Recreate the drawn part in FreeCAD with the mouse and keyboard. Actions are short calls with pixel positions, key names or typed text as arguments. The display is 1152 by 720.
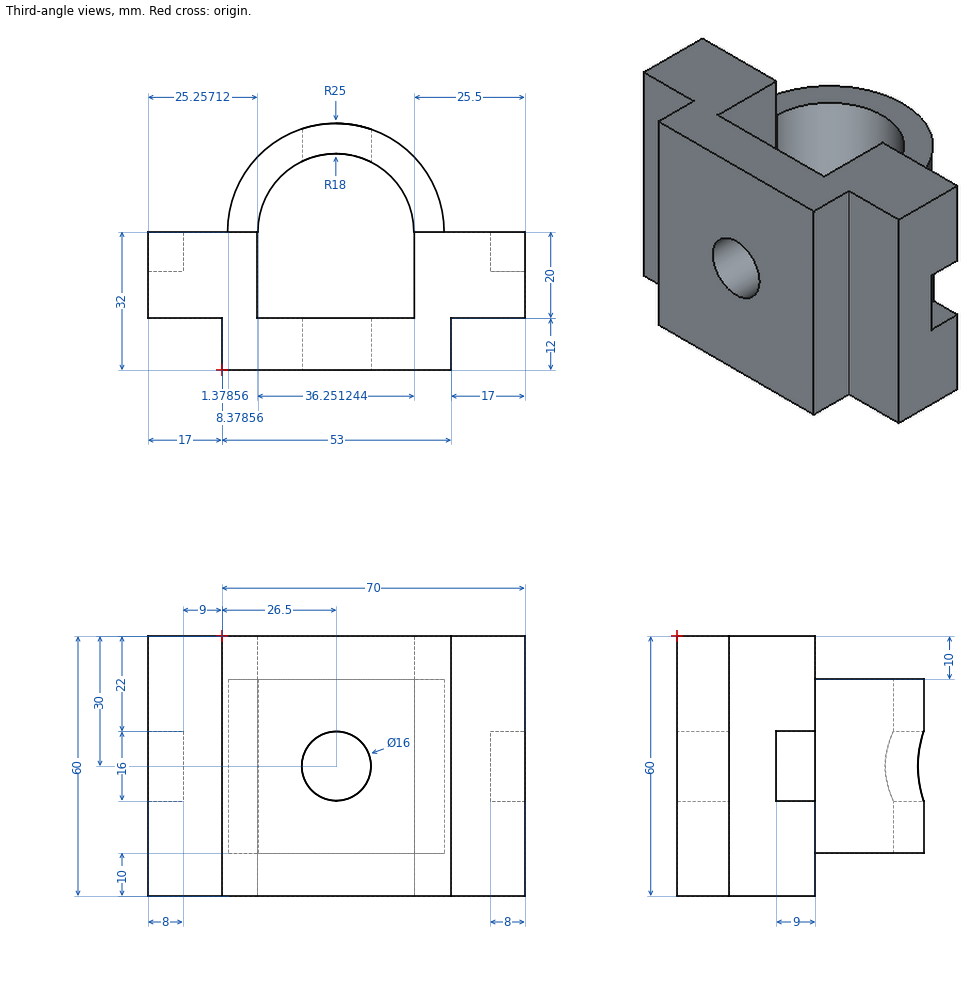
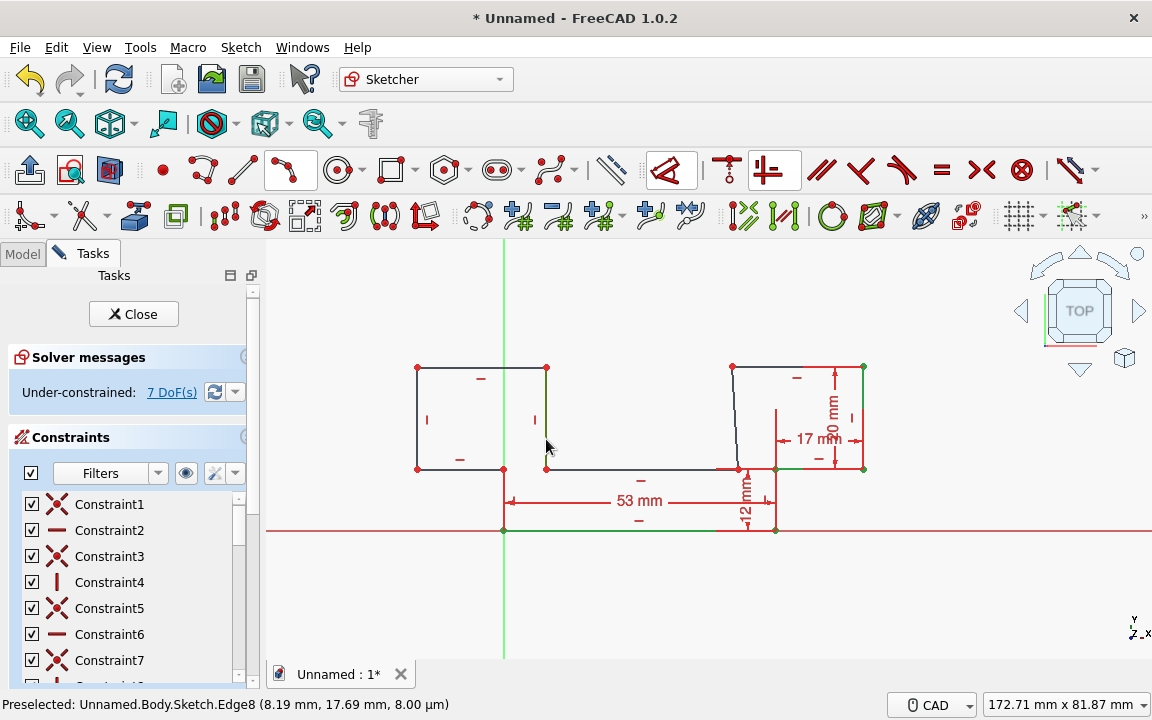
click(692, 170)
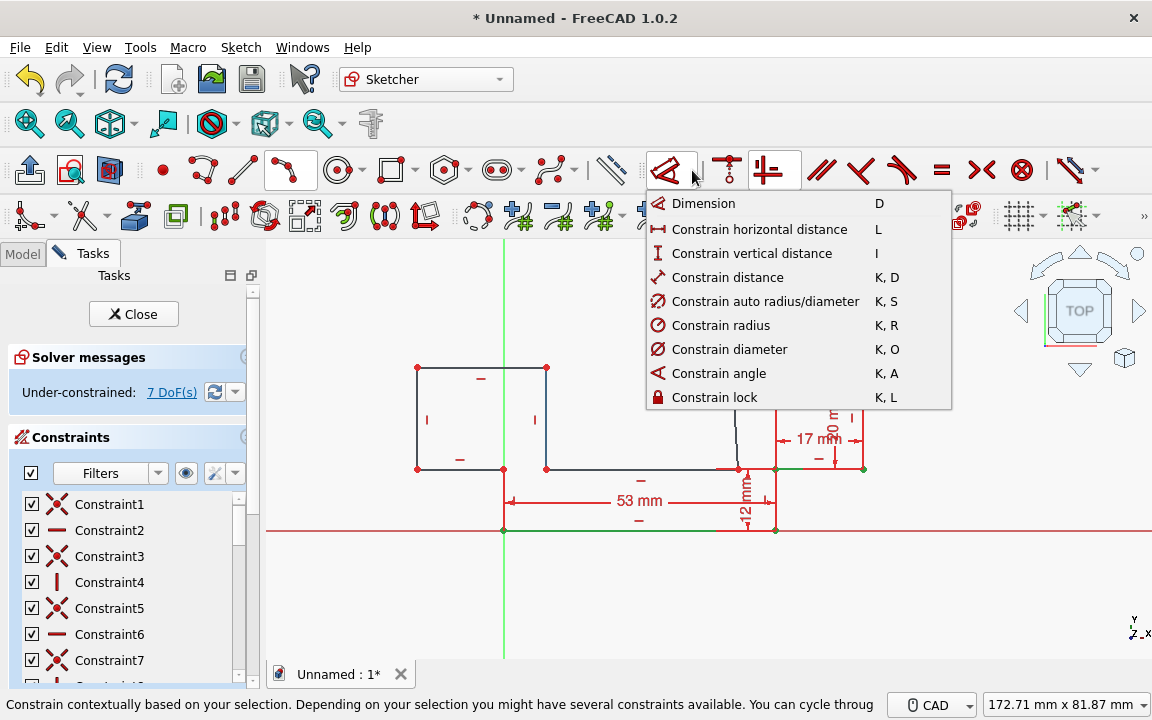
click(799, 253)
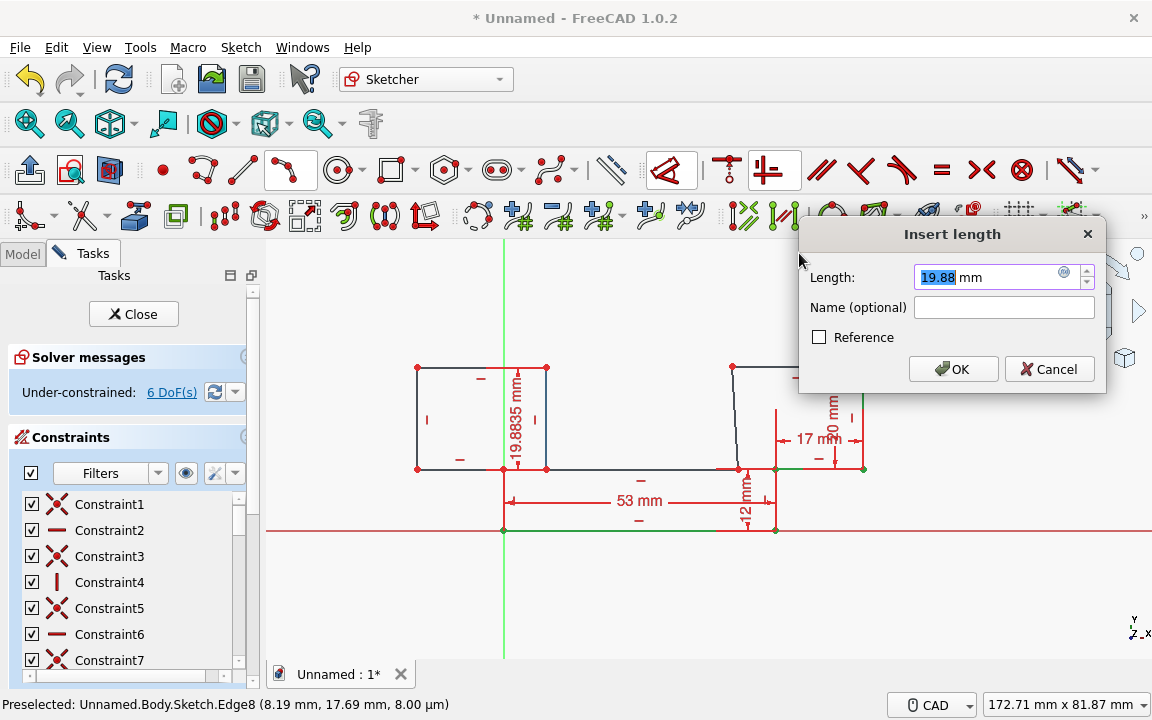
text(20)
key(Return)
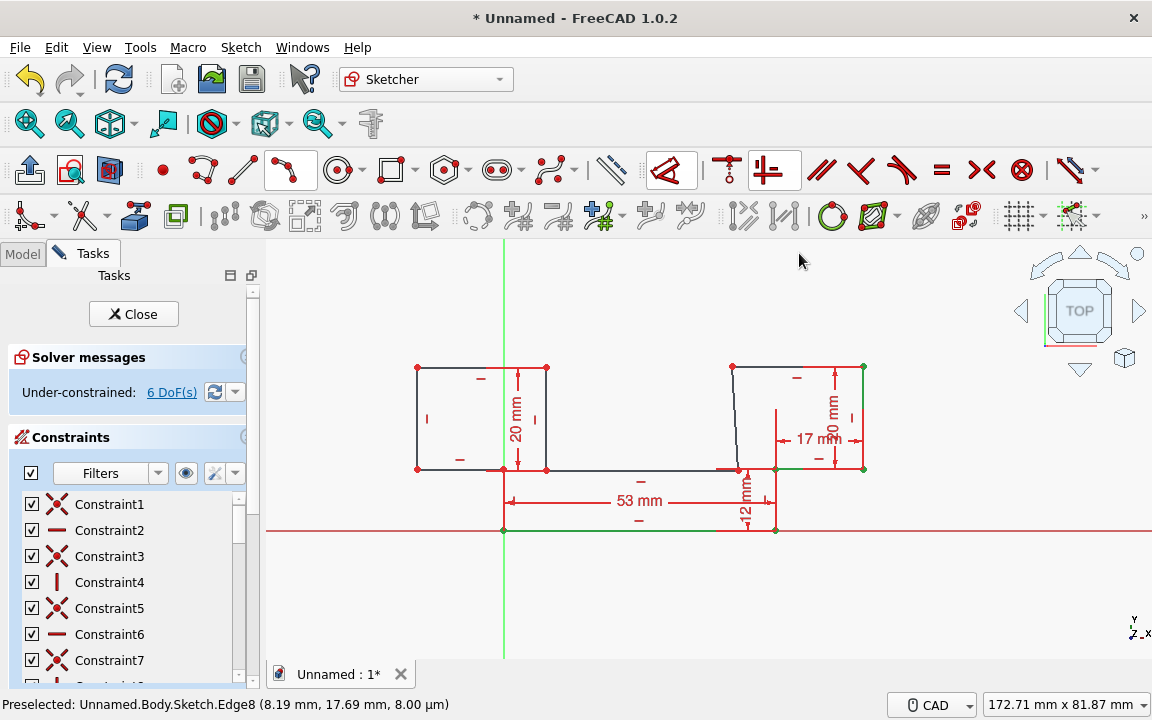
click(417, 399)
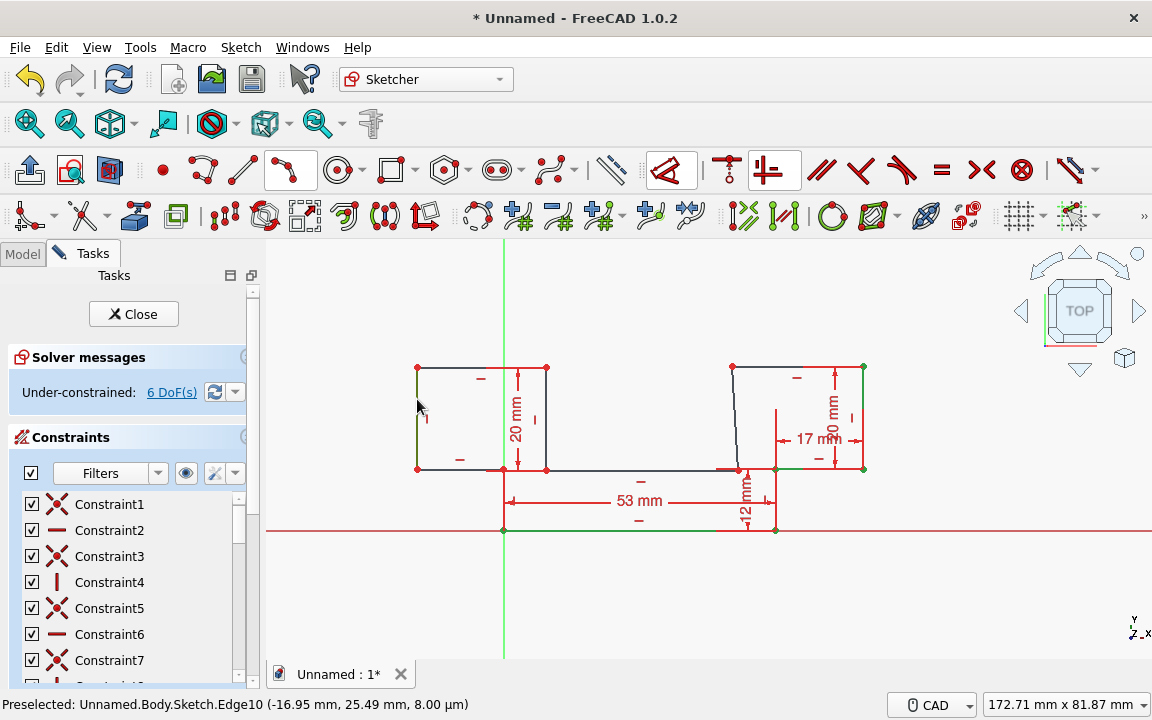
key(i)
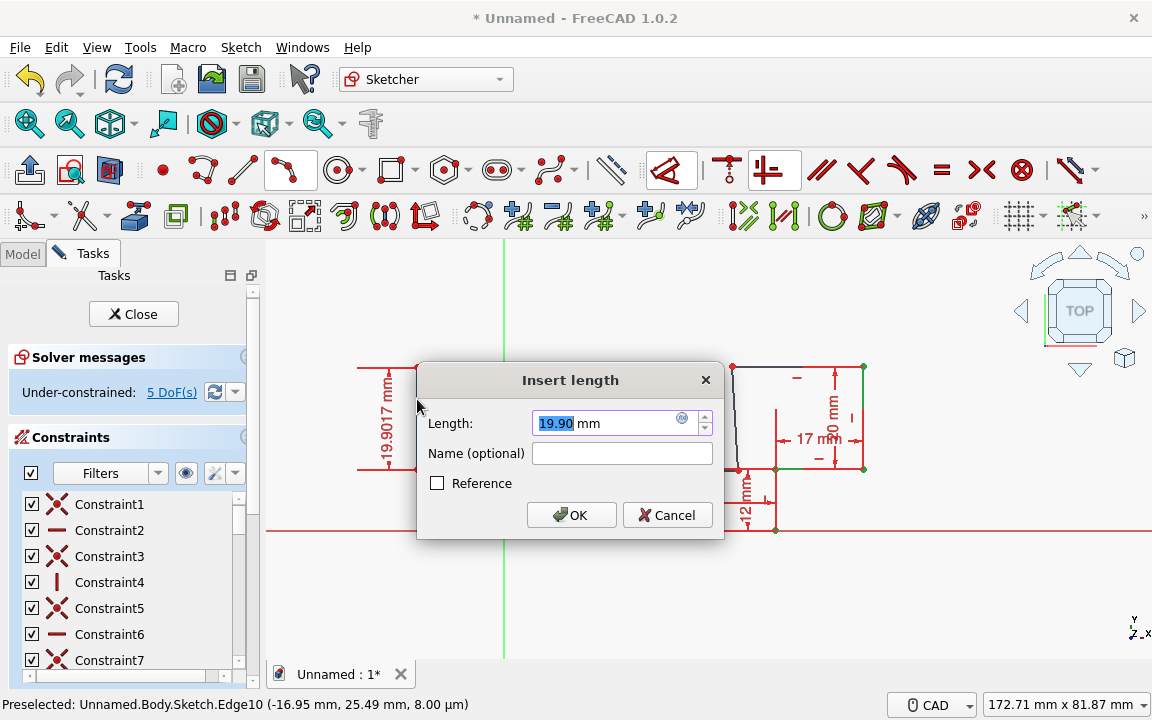
text(20)
key(Return)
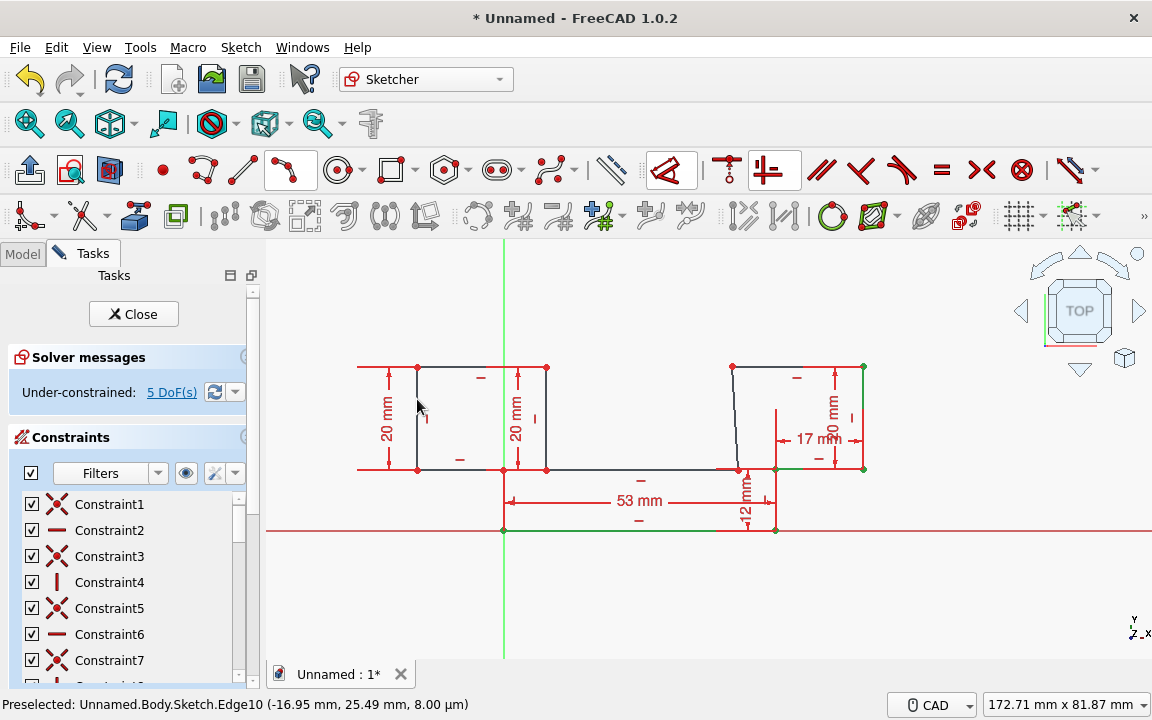
click(443, 470)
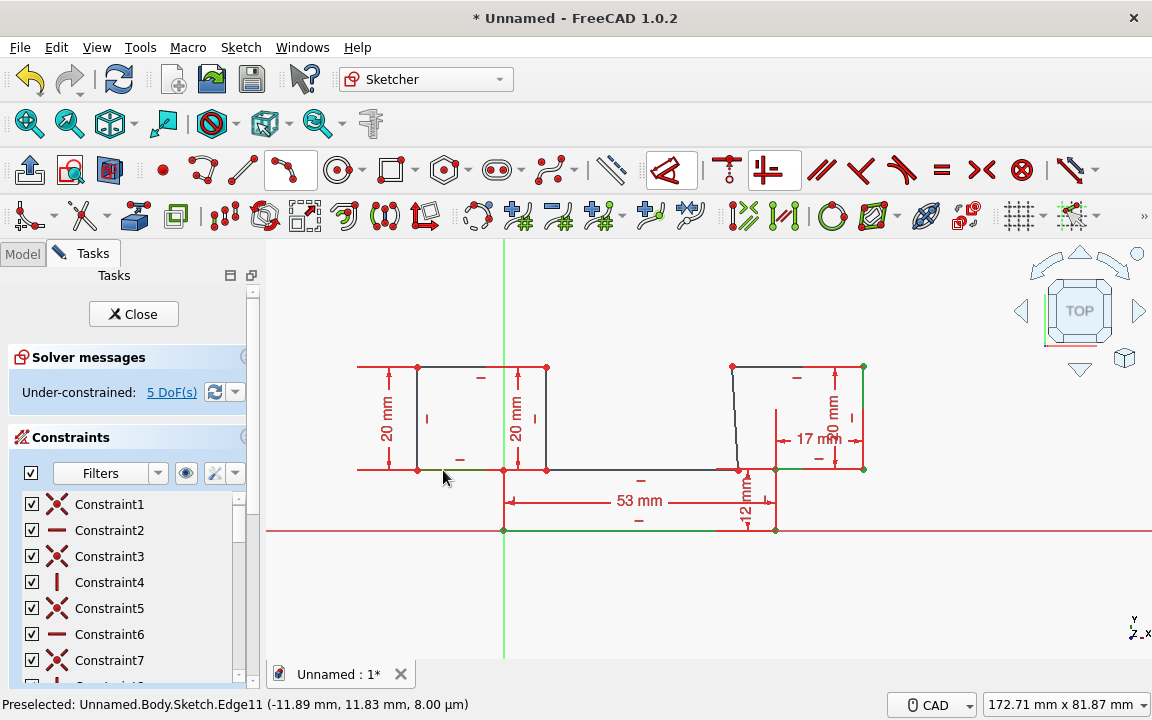
click(692, 170)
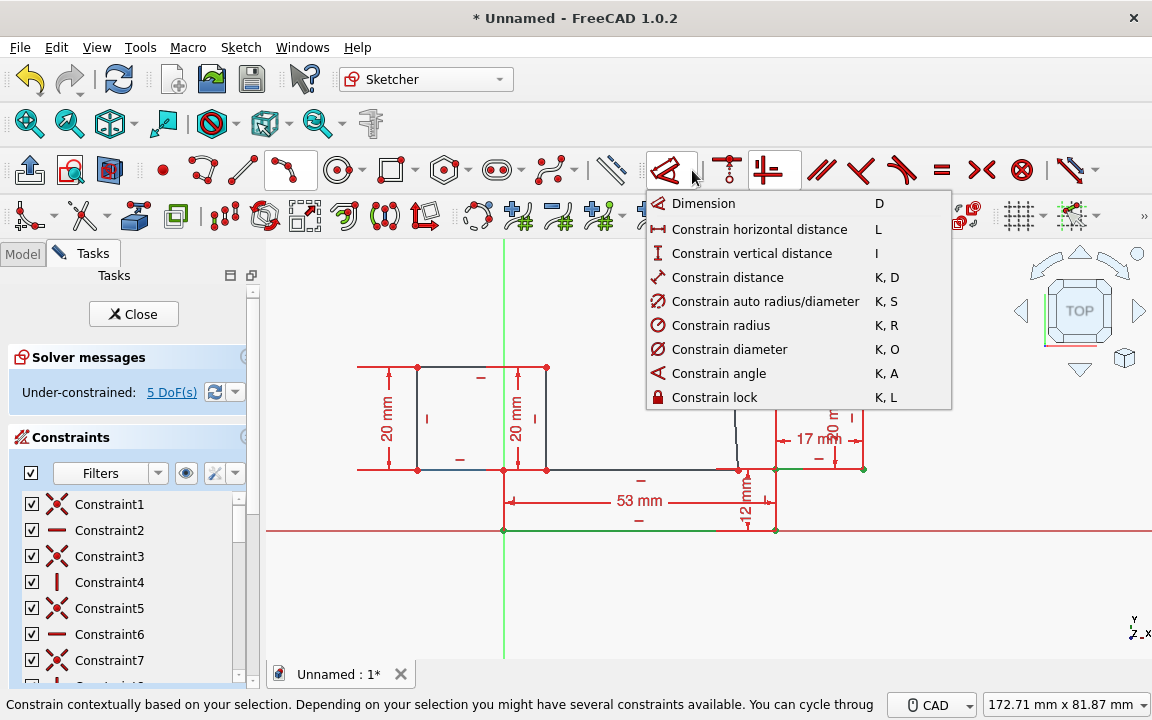
click(799, 229)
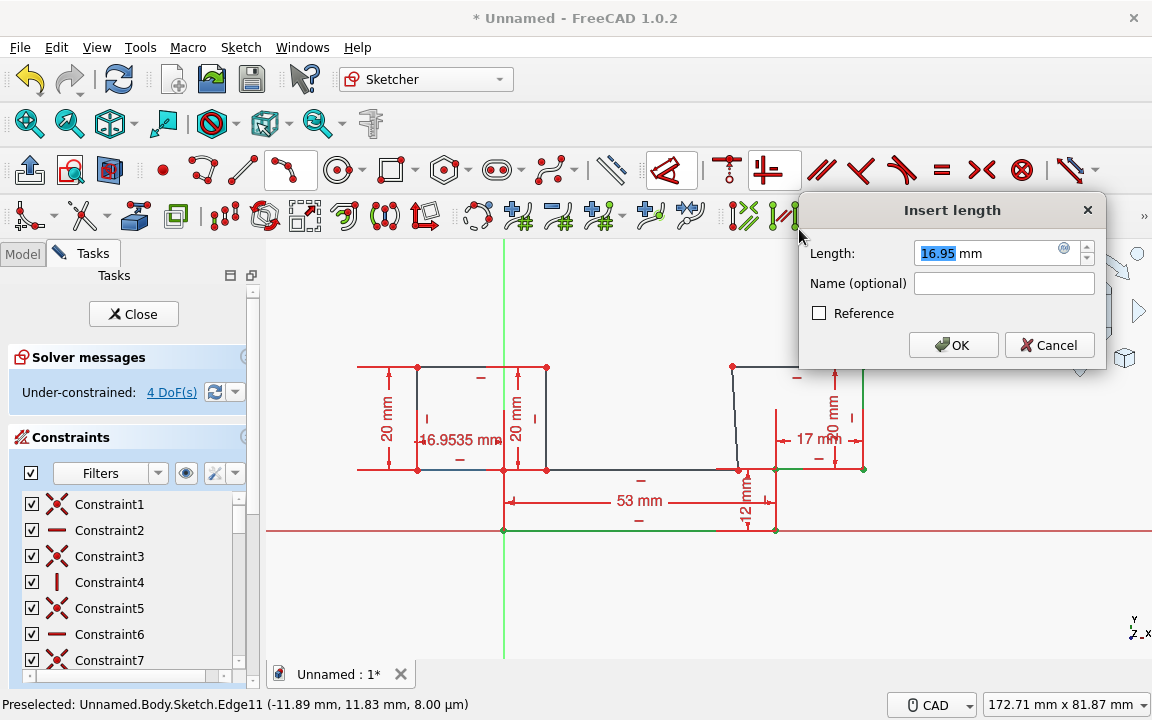
text(17)
key(Return)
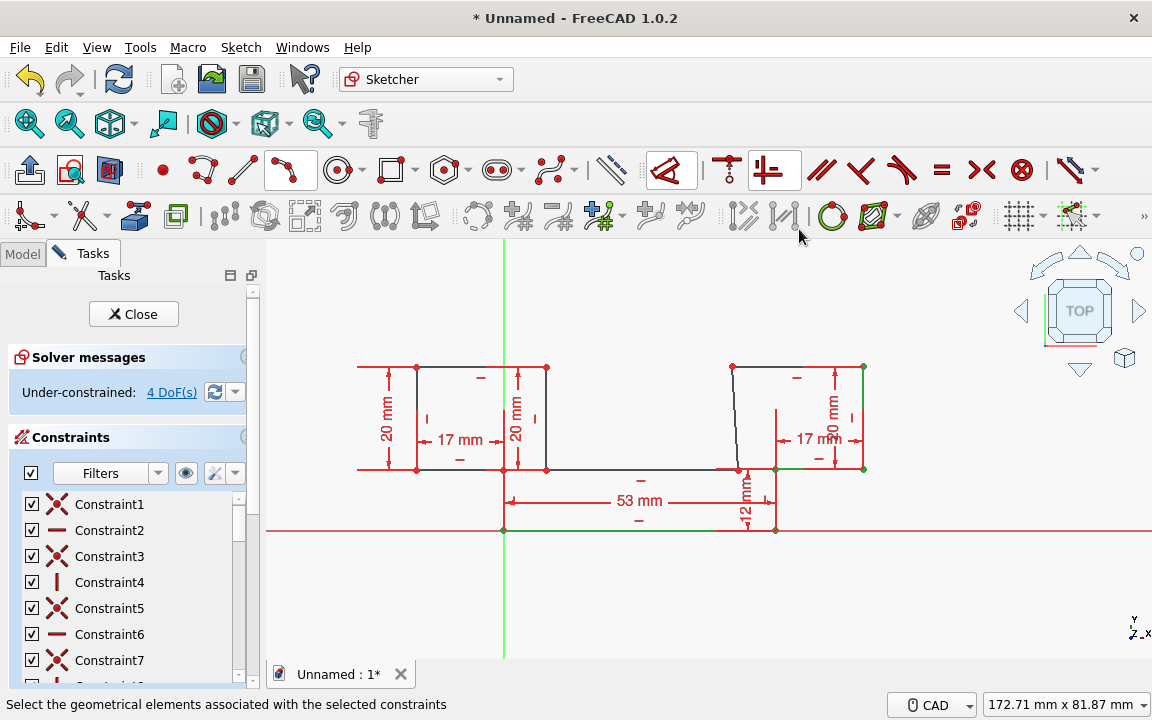
click(504, 488)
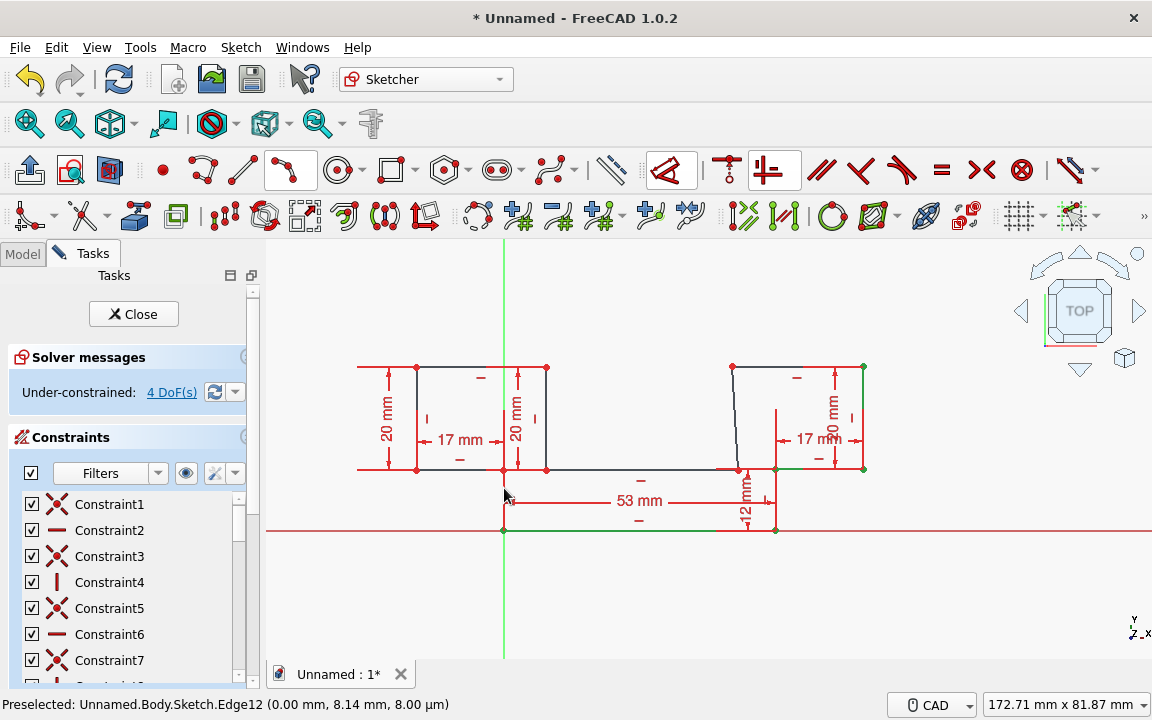
key(i)